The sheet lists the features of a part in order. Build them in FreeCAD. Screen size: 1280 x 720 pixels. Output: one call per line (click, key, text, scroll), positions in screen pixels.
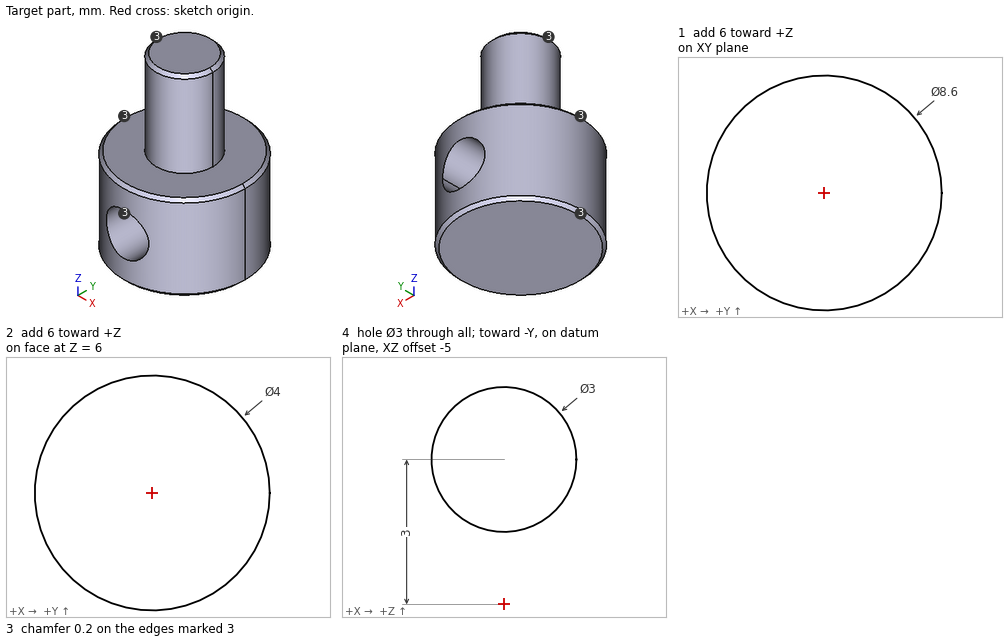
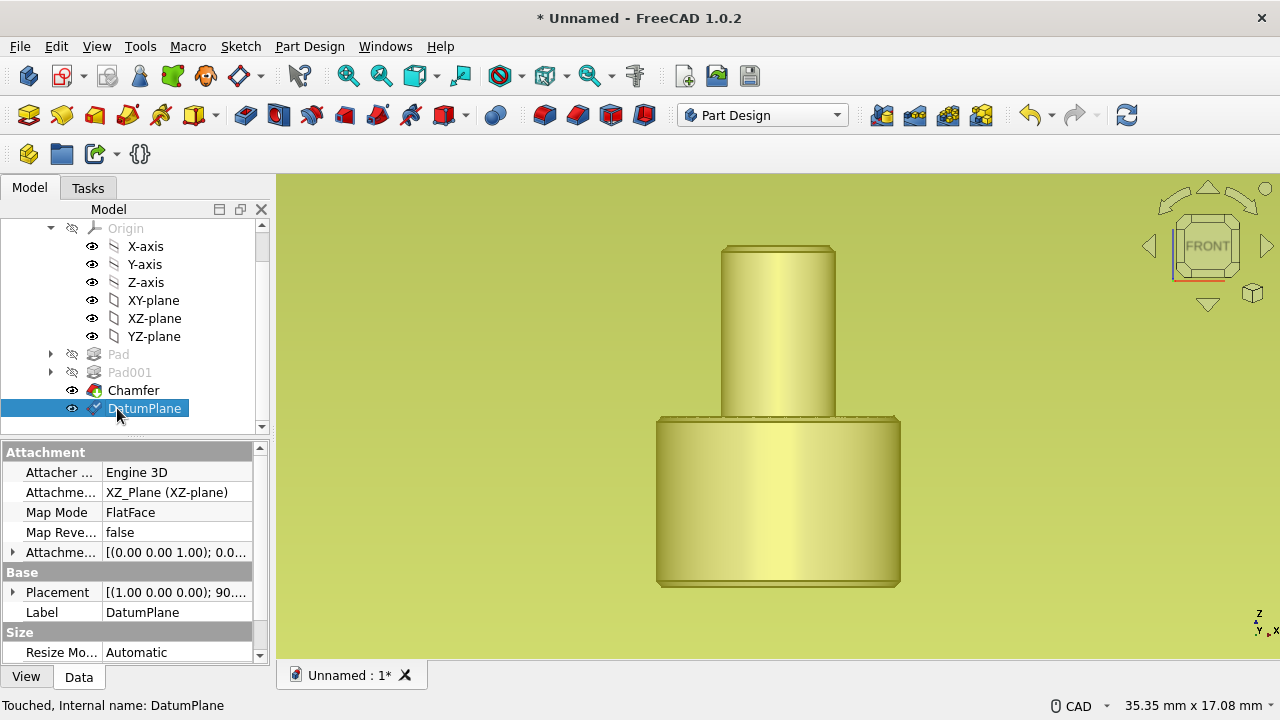
click(62, 76)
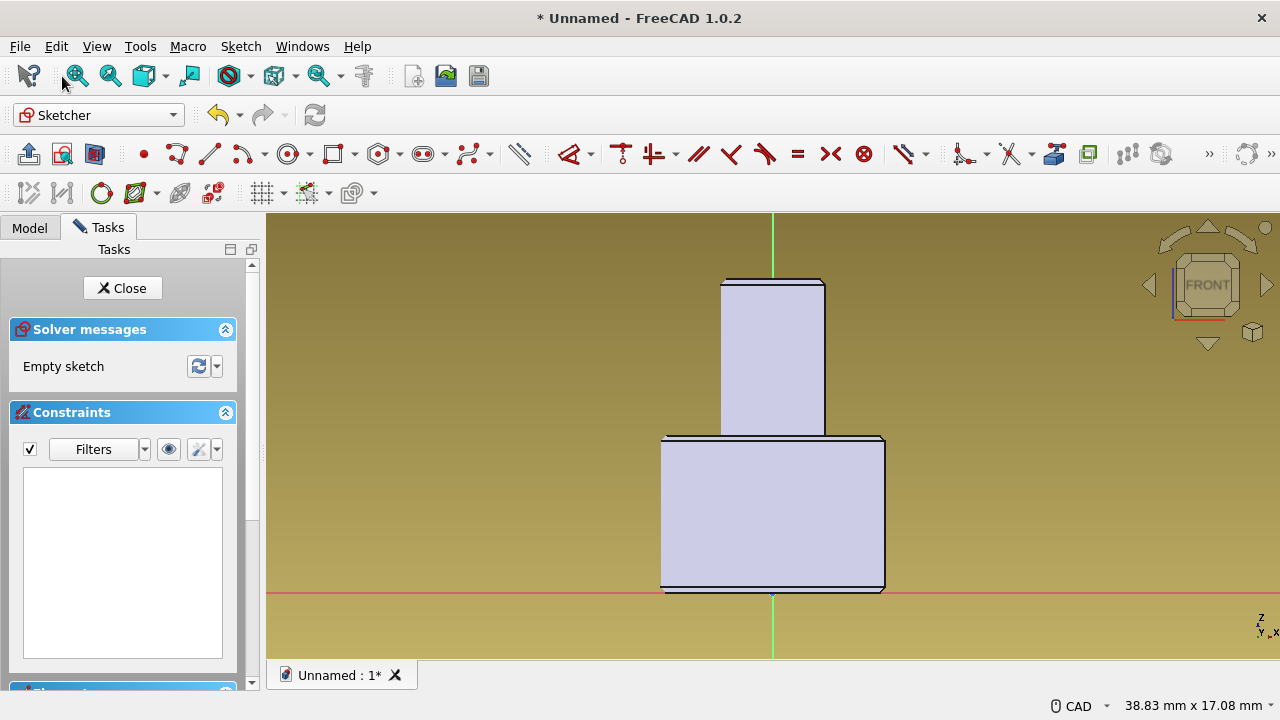
click(95, 154)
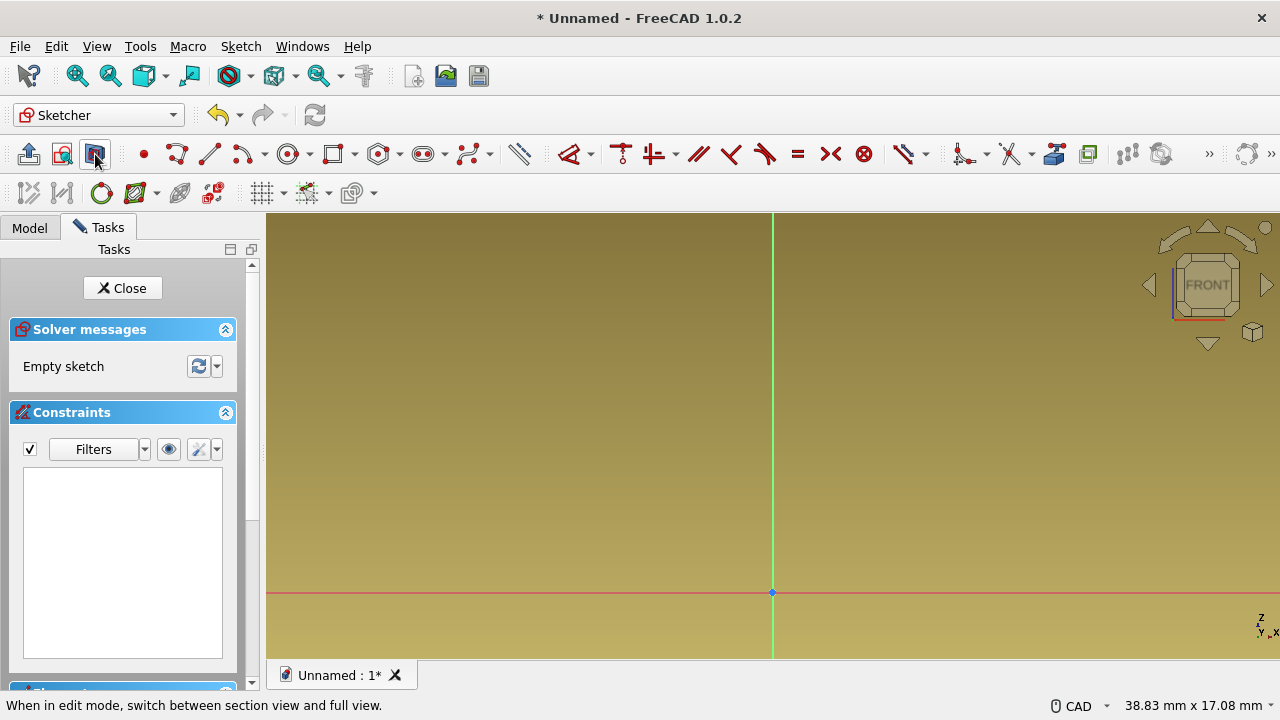
scroll(829, 614, up, 4)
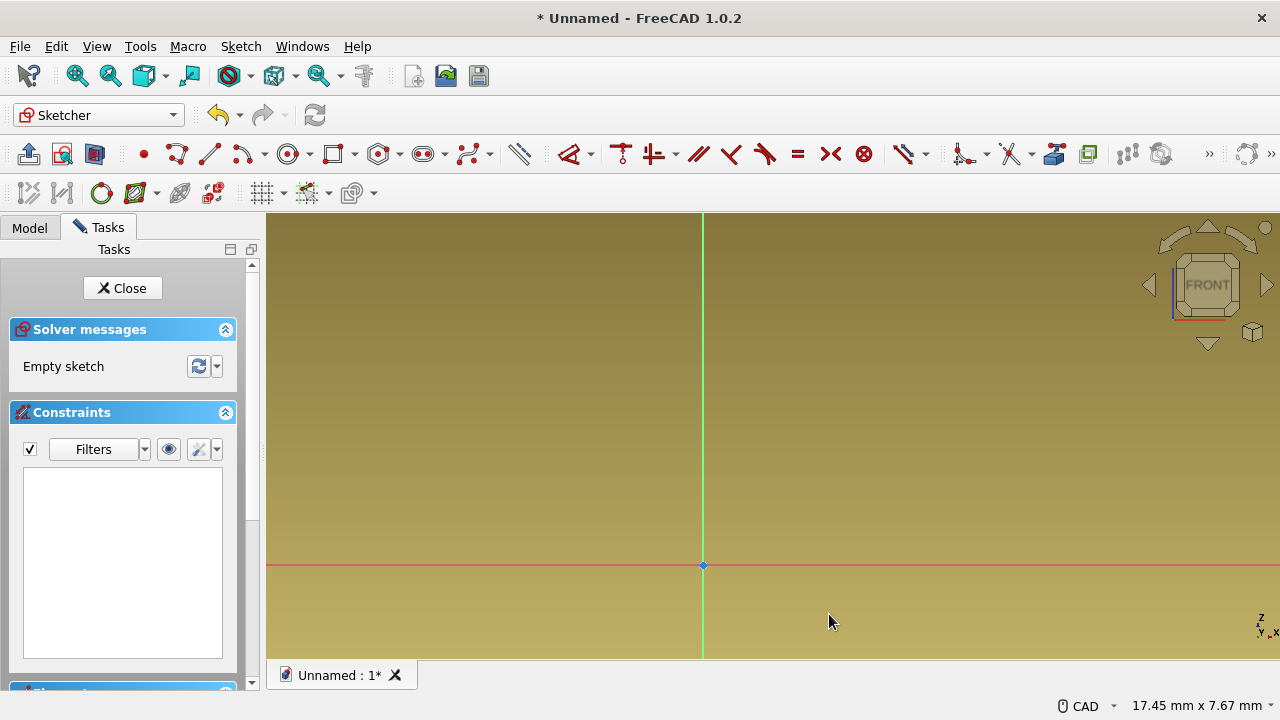
click(288, 154)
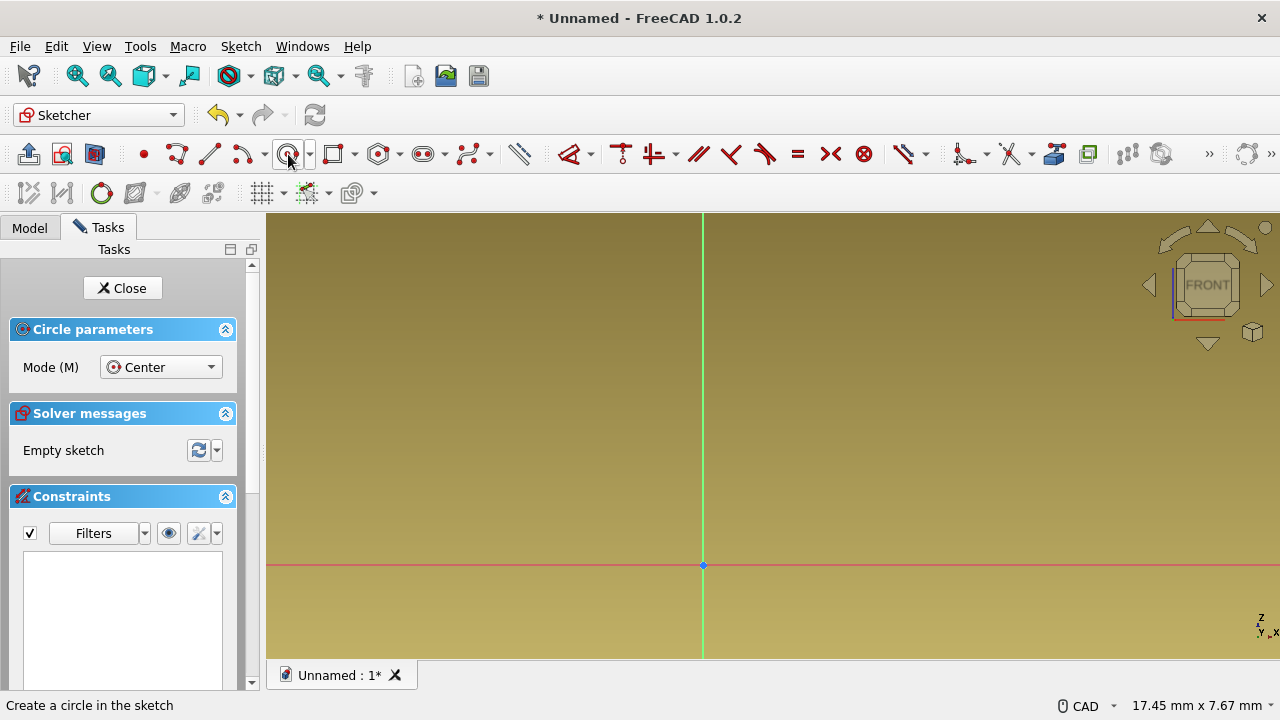
click(703, 391)
move(765, 329)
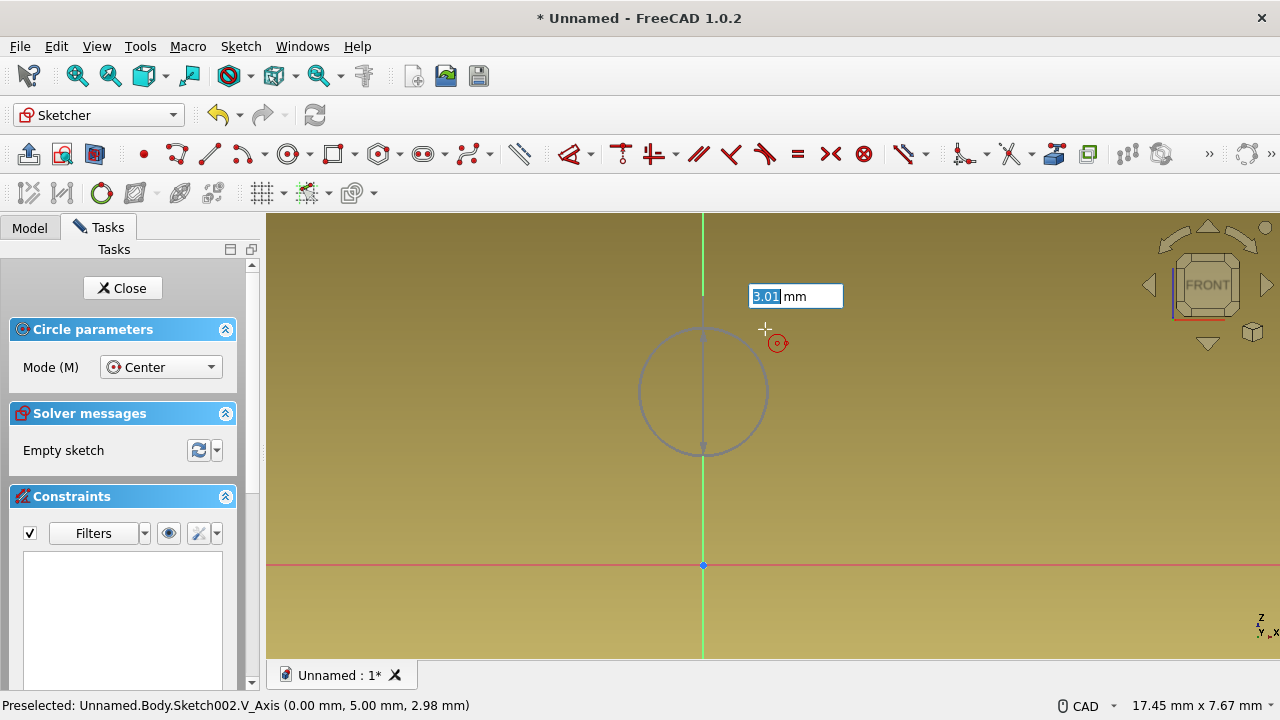
text(3)
key(Return)
key(Escape)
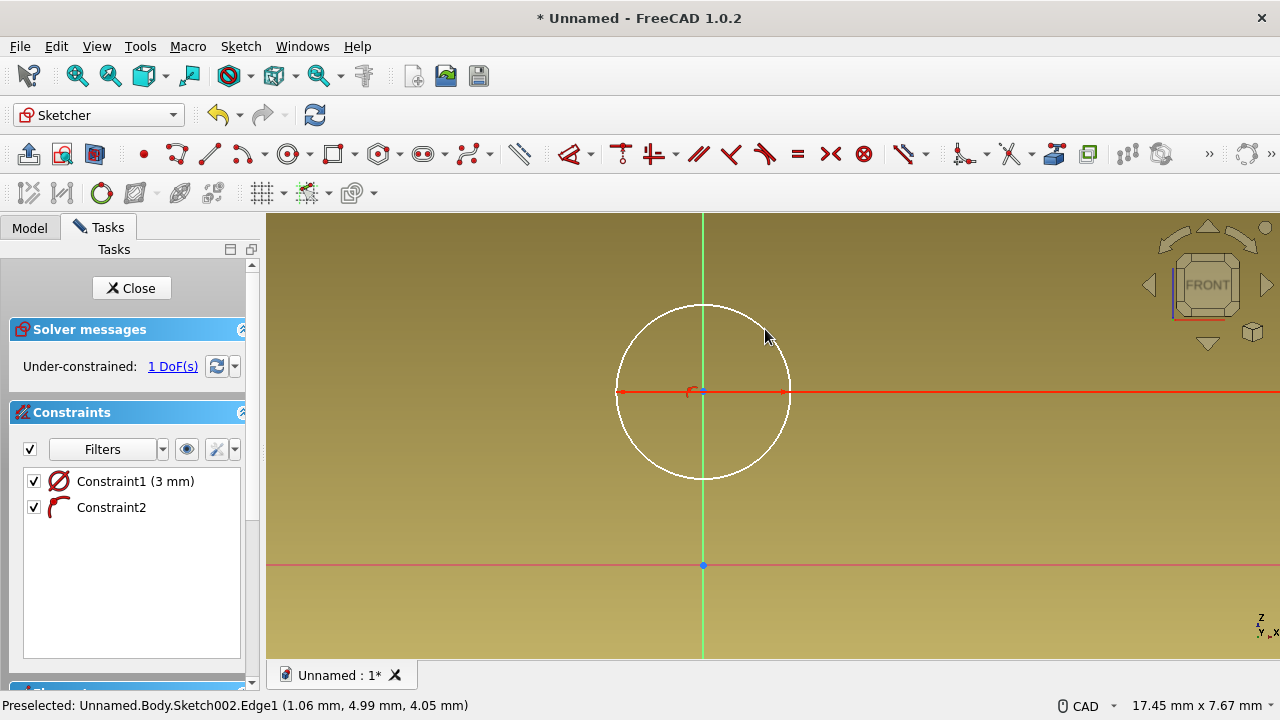
click(568, 154)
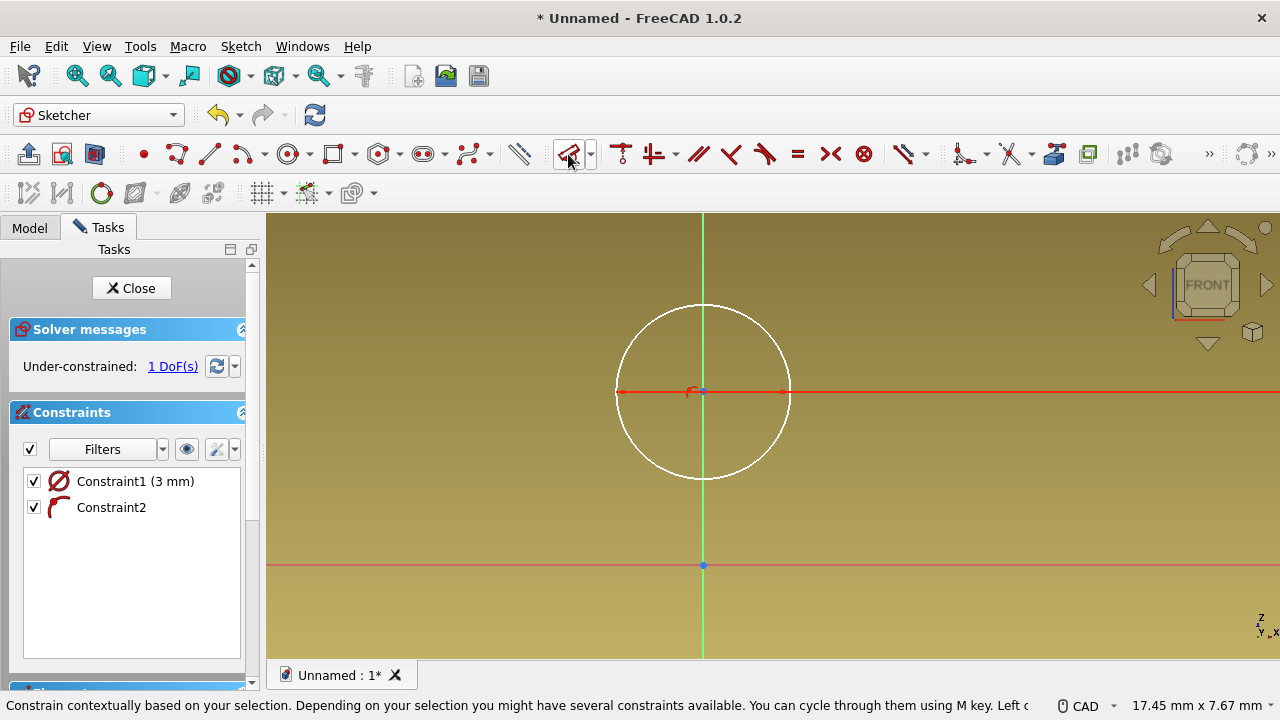
click(703, 392)
click(737, 439)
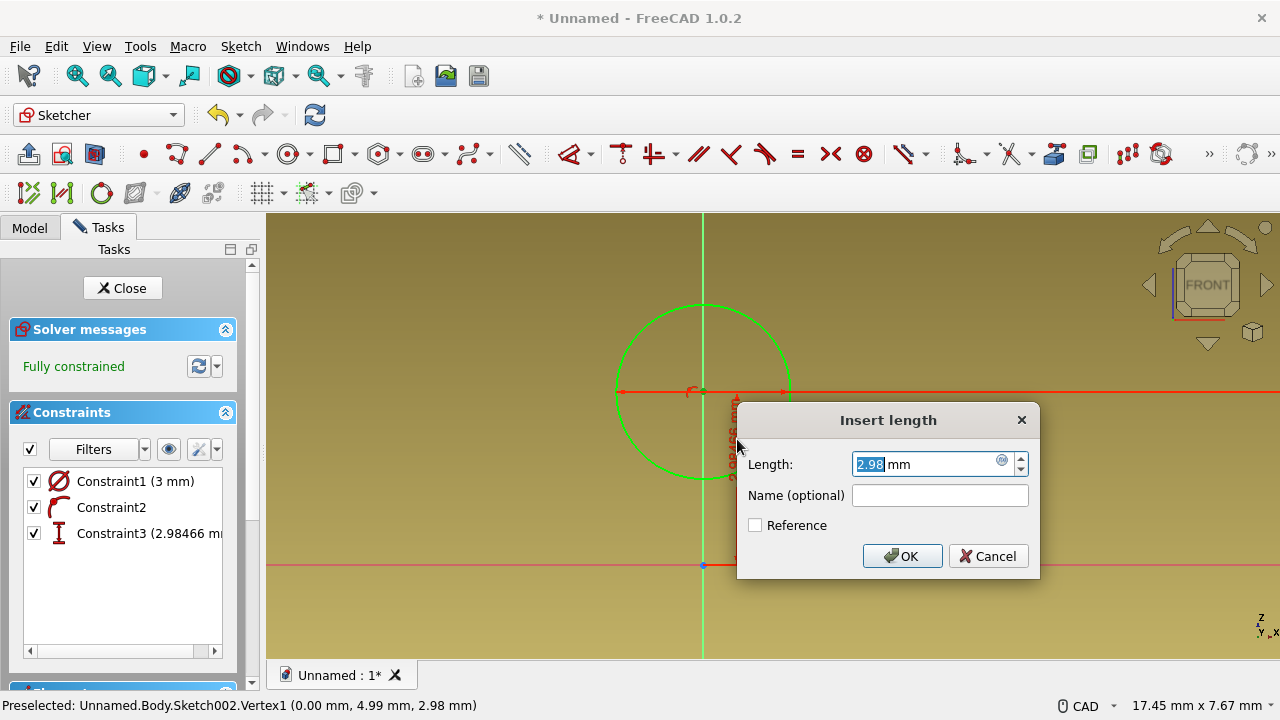
text(3)
key(Return)
key(Escape)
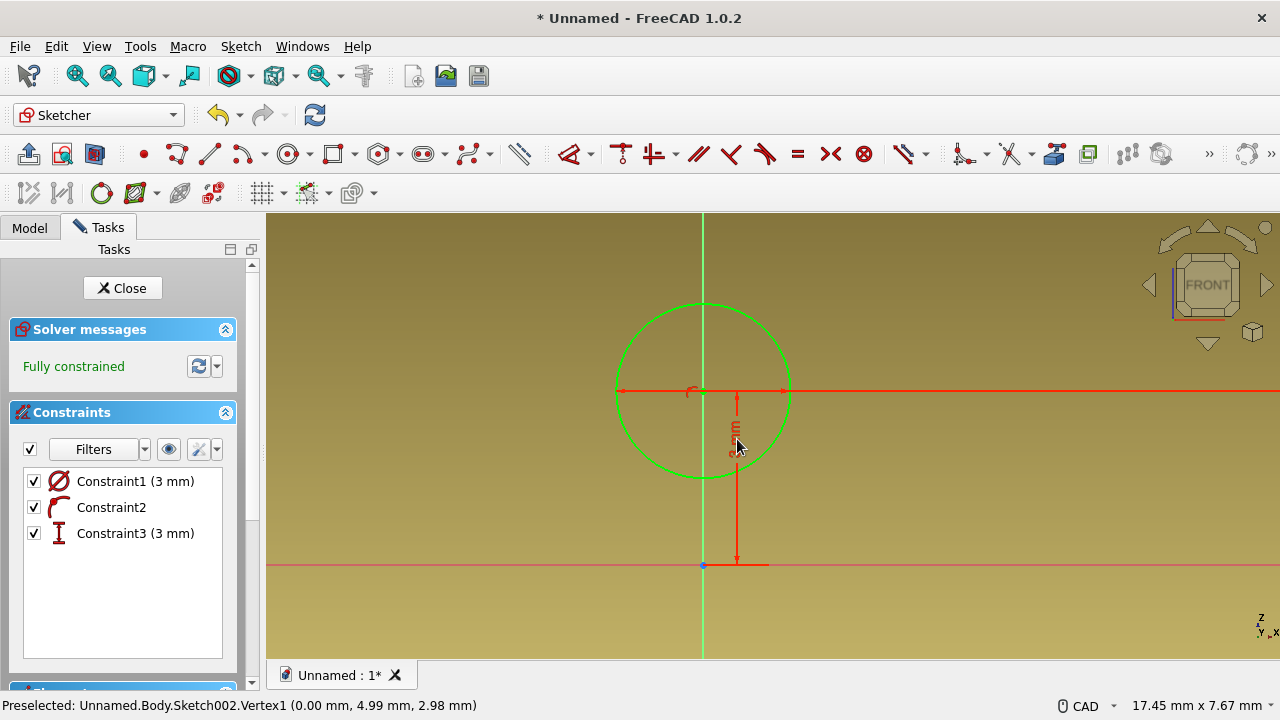
click(123, 288)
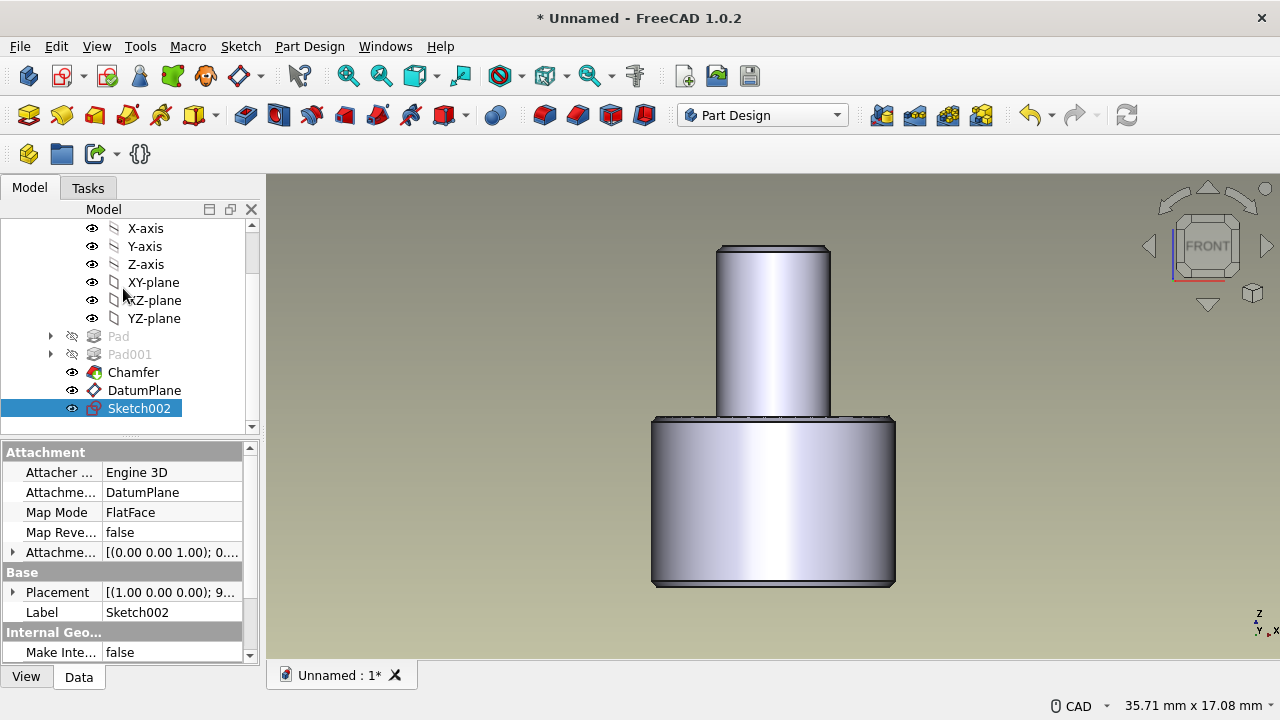
click(279, 116)